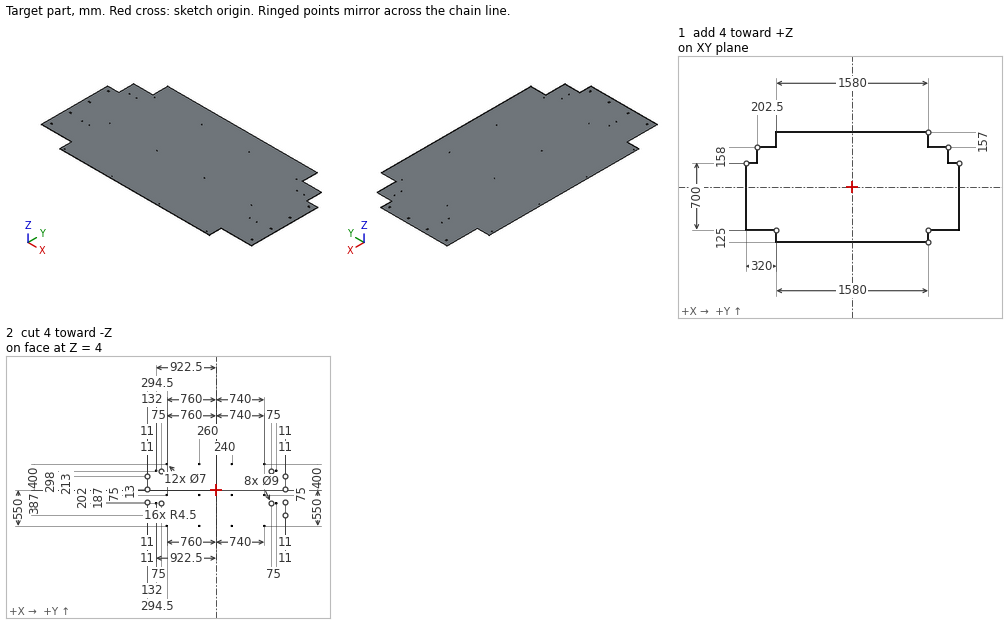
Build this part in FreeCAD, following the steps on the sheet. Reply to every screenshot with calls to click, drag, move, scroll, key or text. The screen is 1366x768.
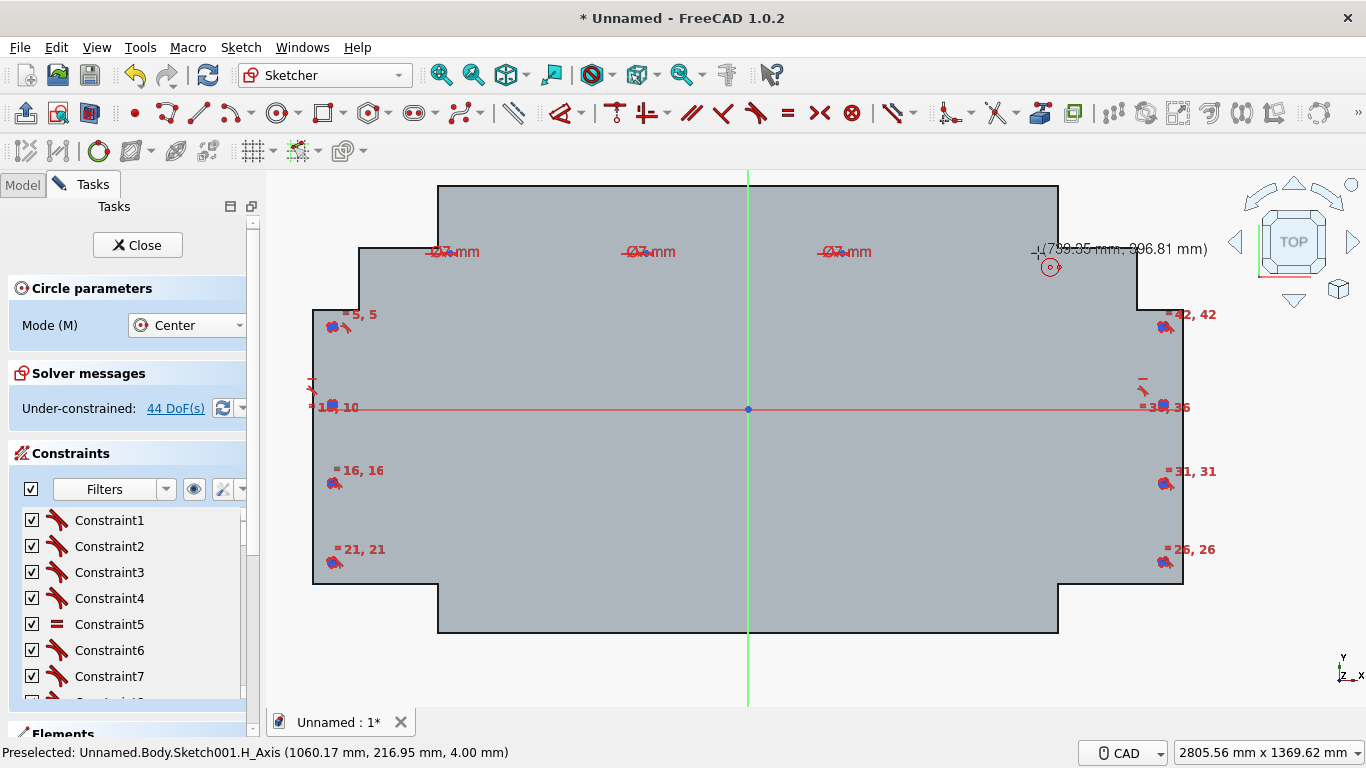
click(1038, 253)
move(1039, 252)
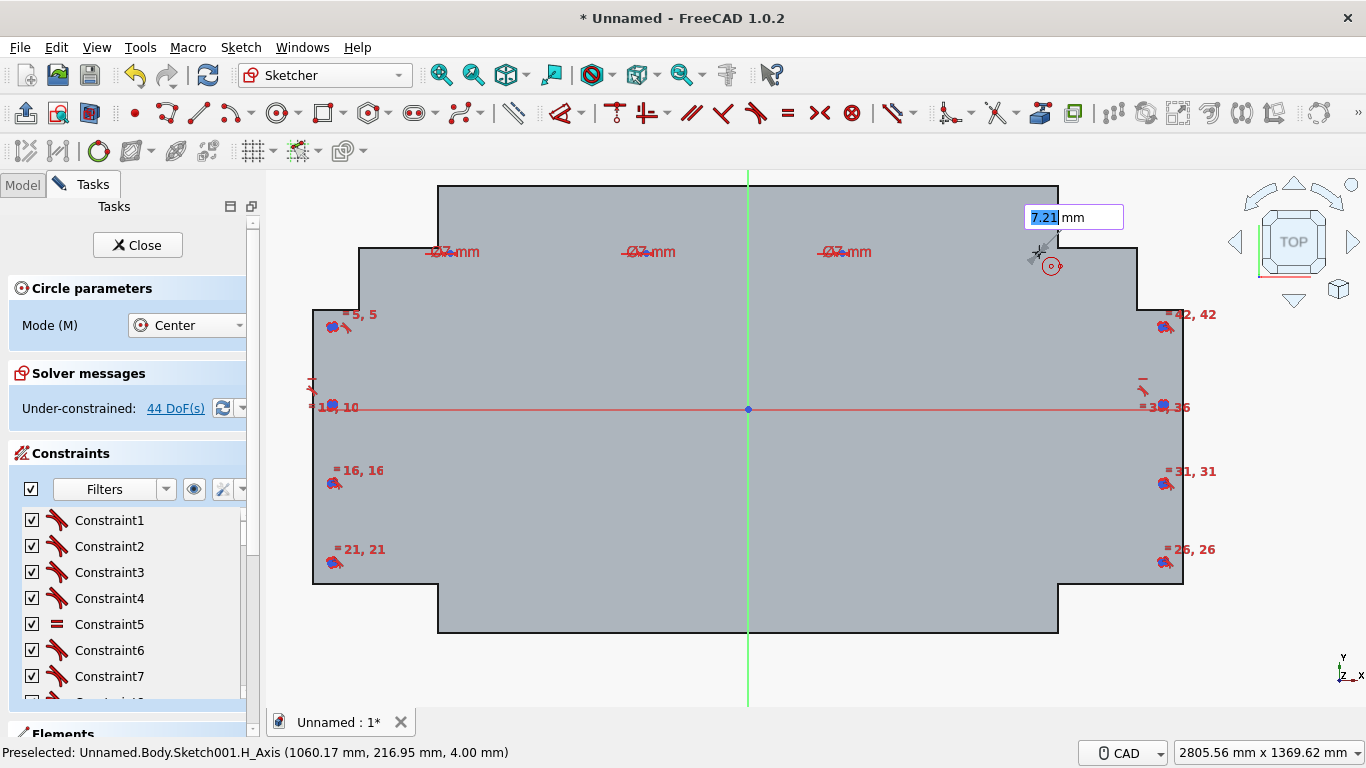
text(7)
key(Return)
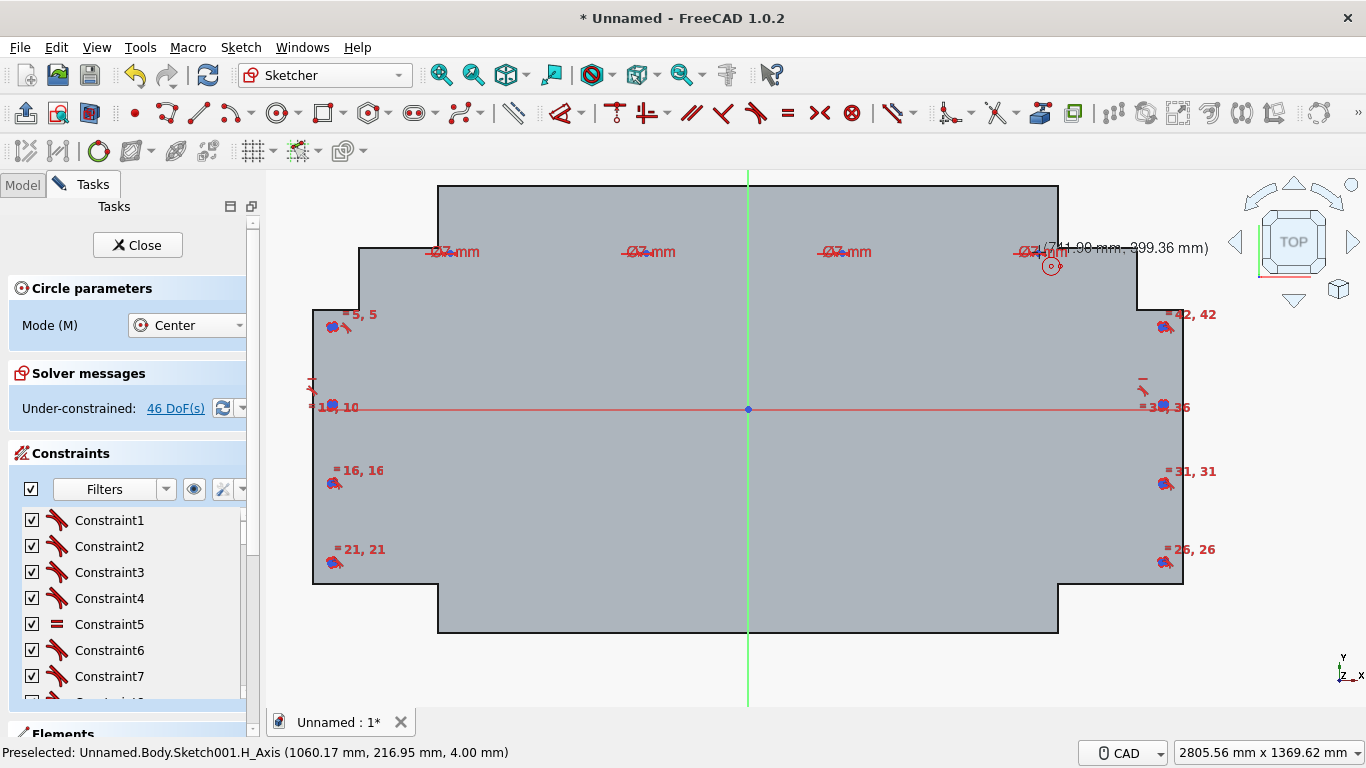
scroll(450, 439, up, 15)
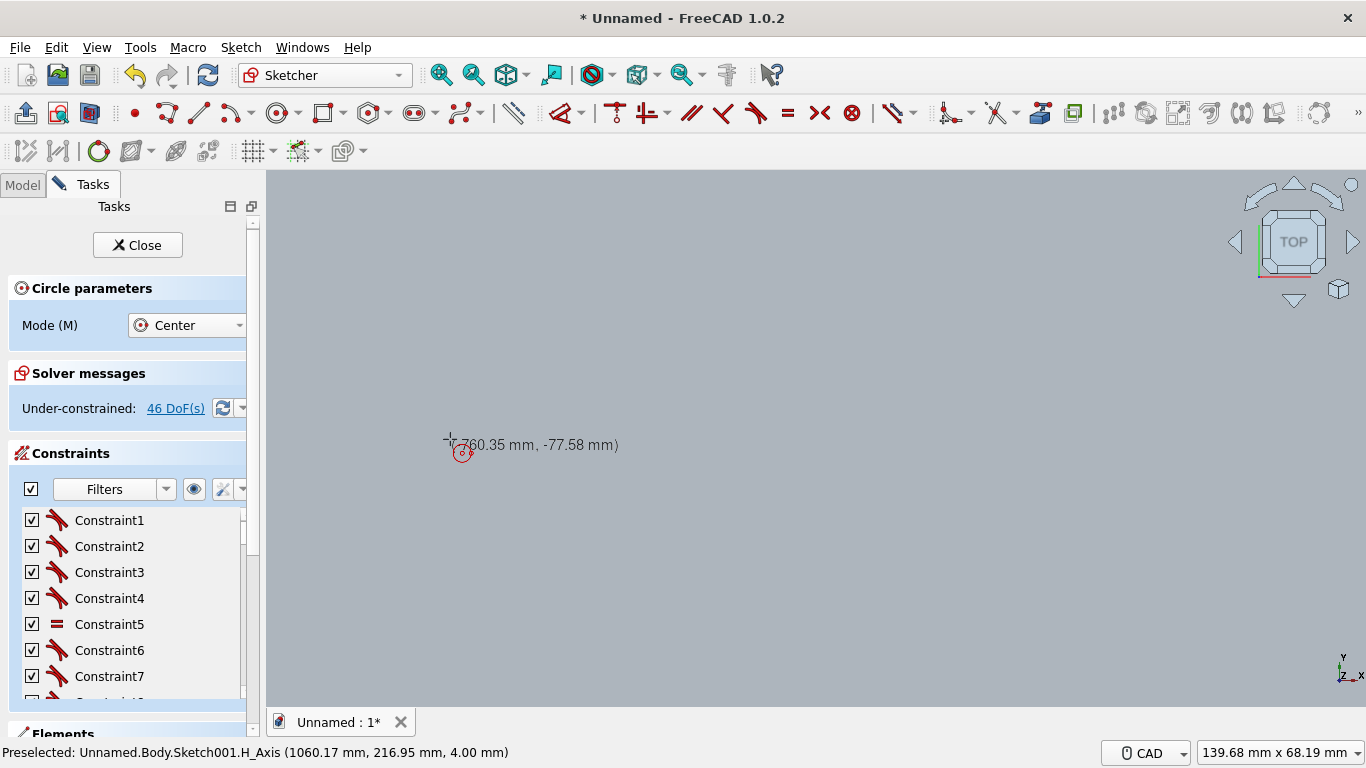
scroll(450, 439, down, 15)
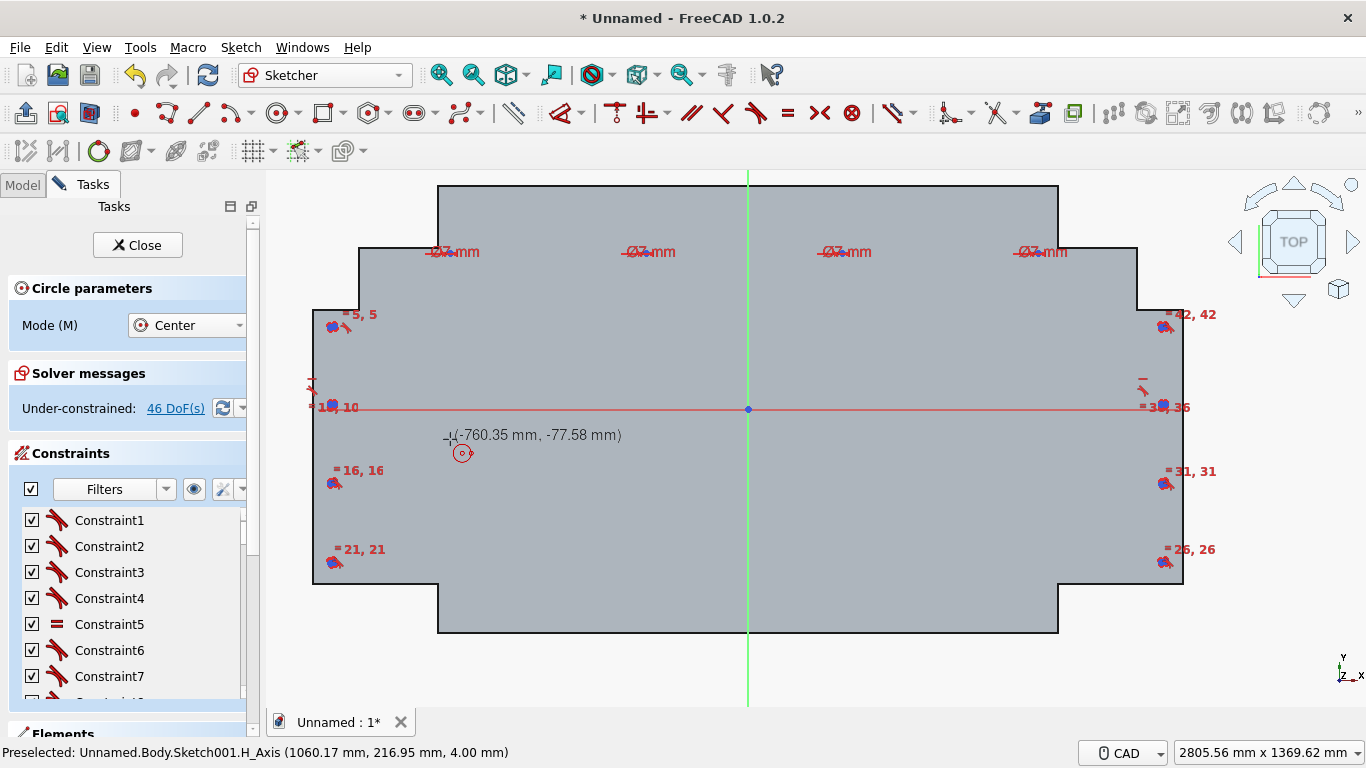
click(450, 439)
move(451, 438)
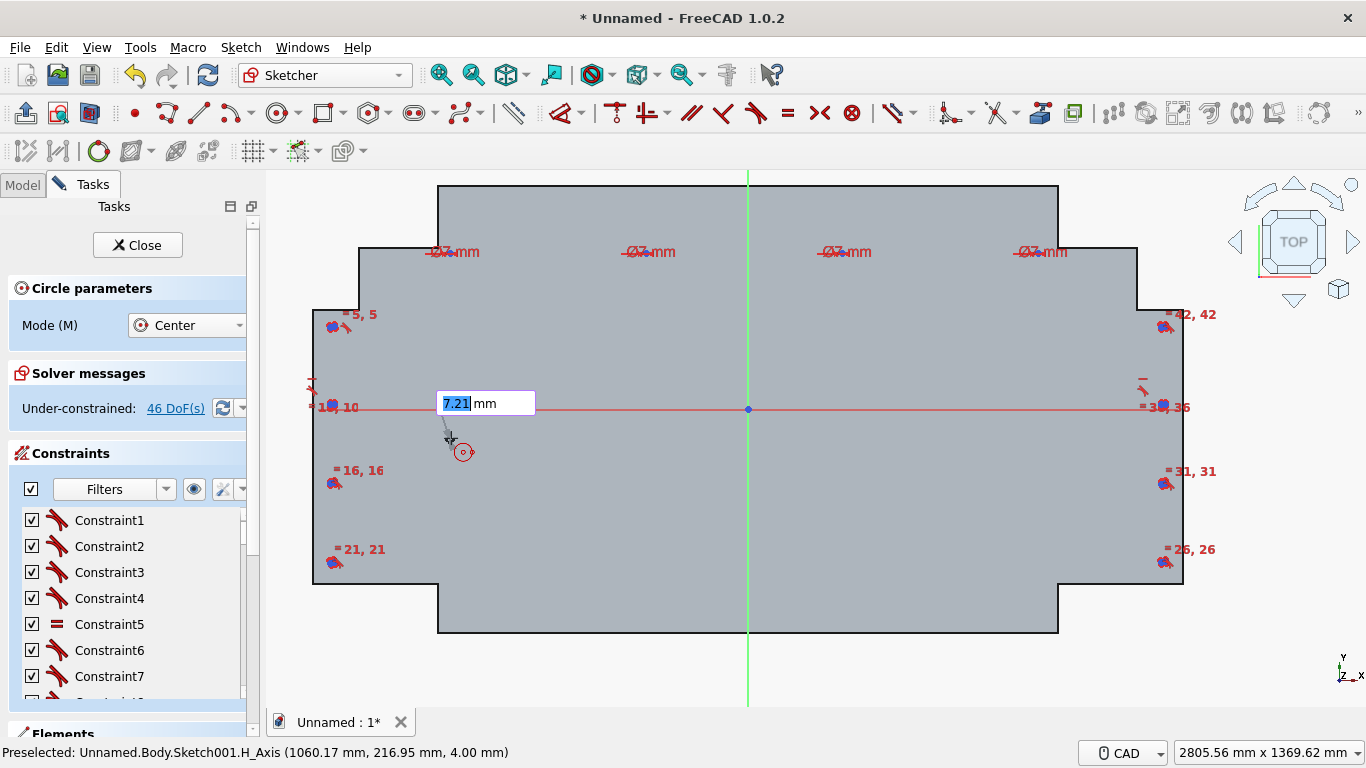
text(7)
key(Return)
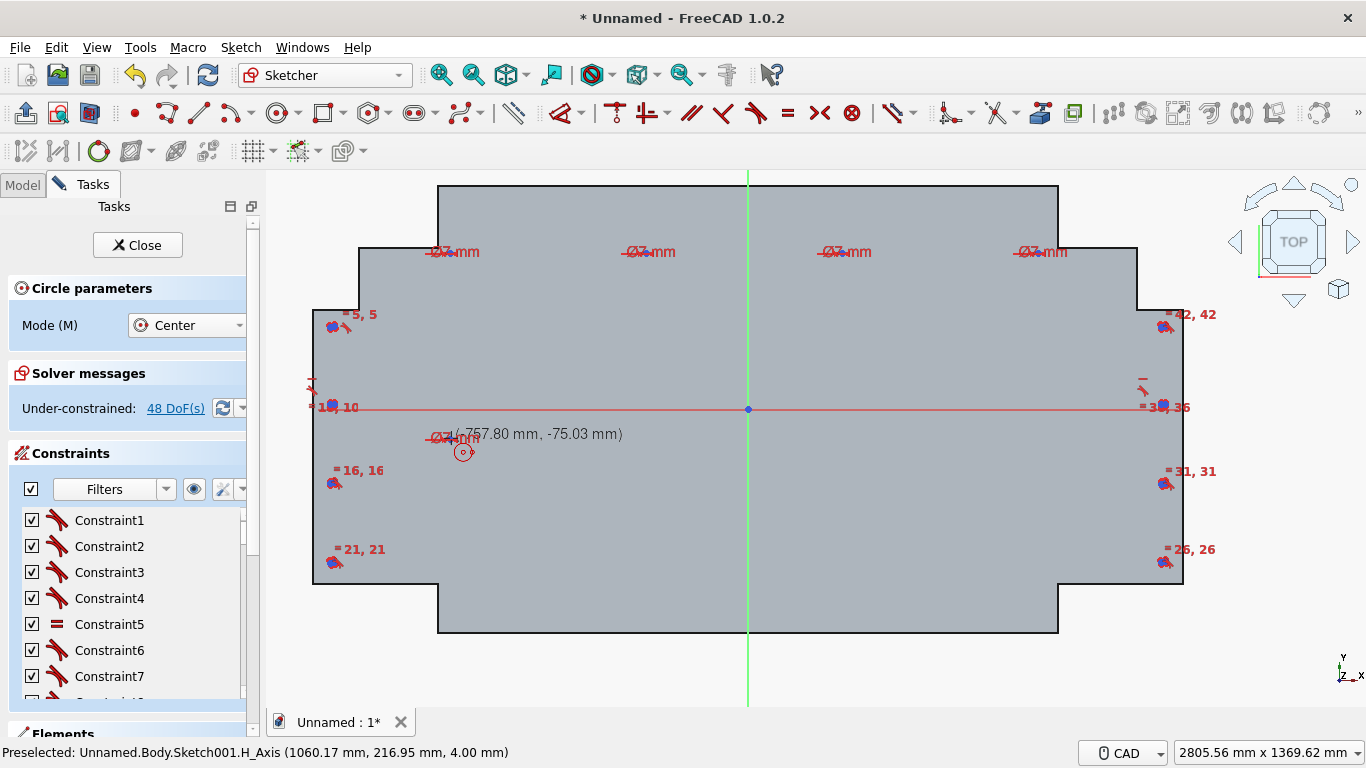
scroll(646, 439, up, 15)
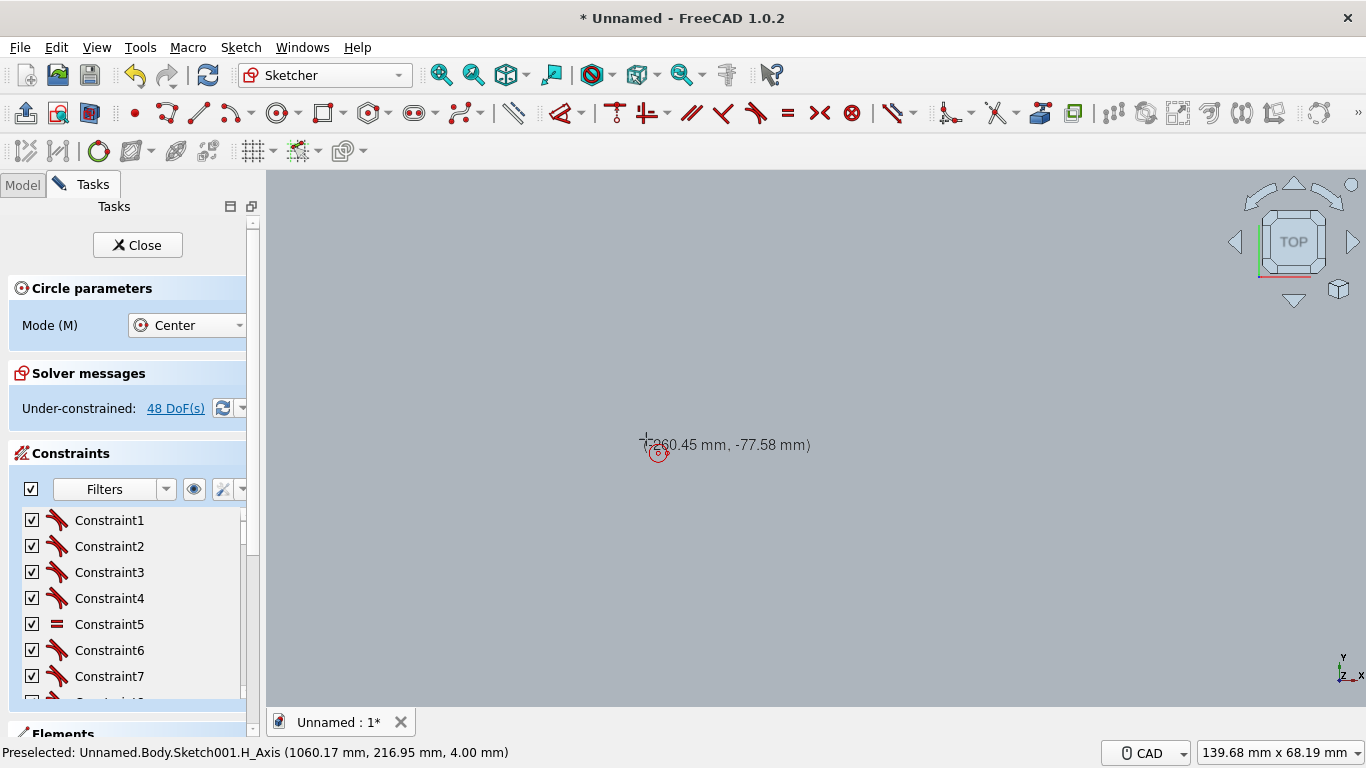
scroll(646, 439, down, 15)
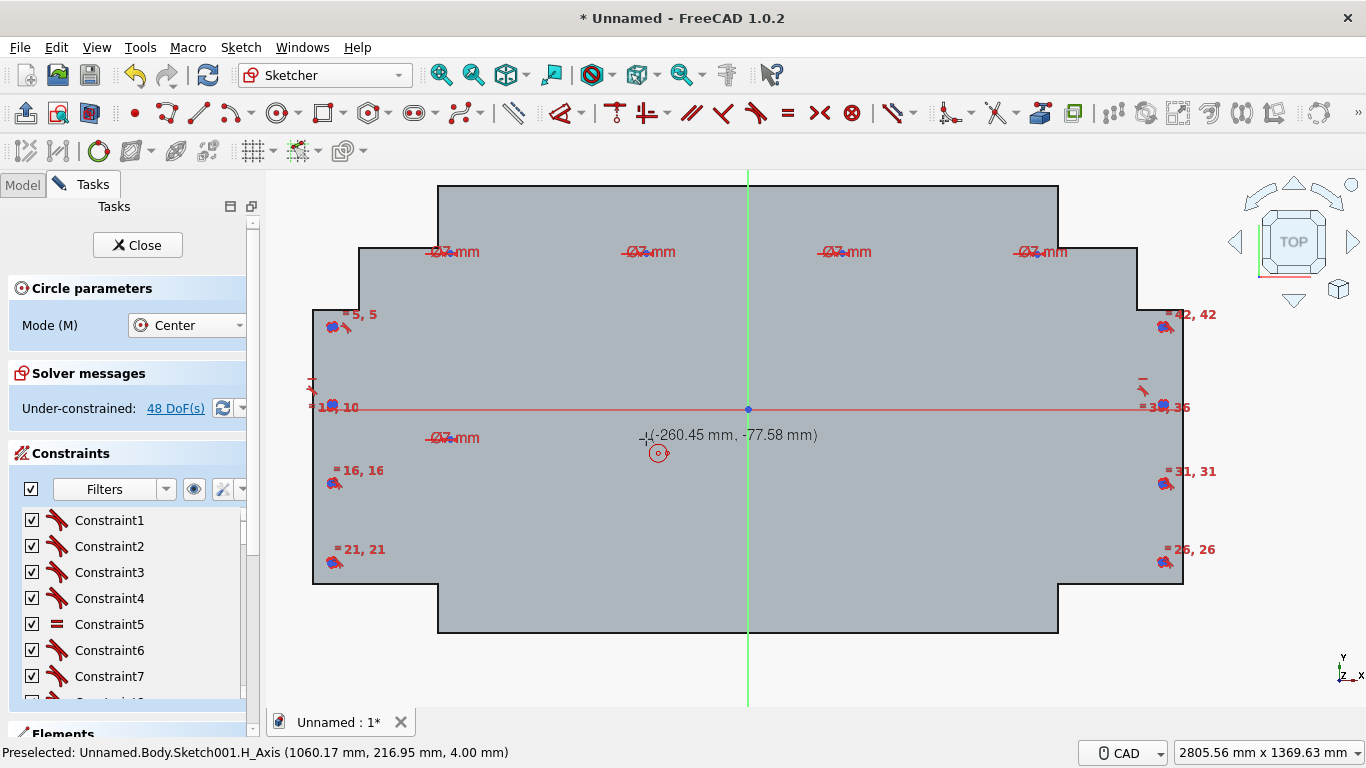
click(646, 439)
move(647, 438)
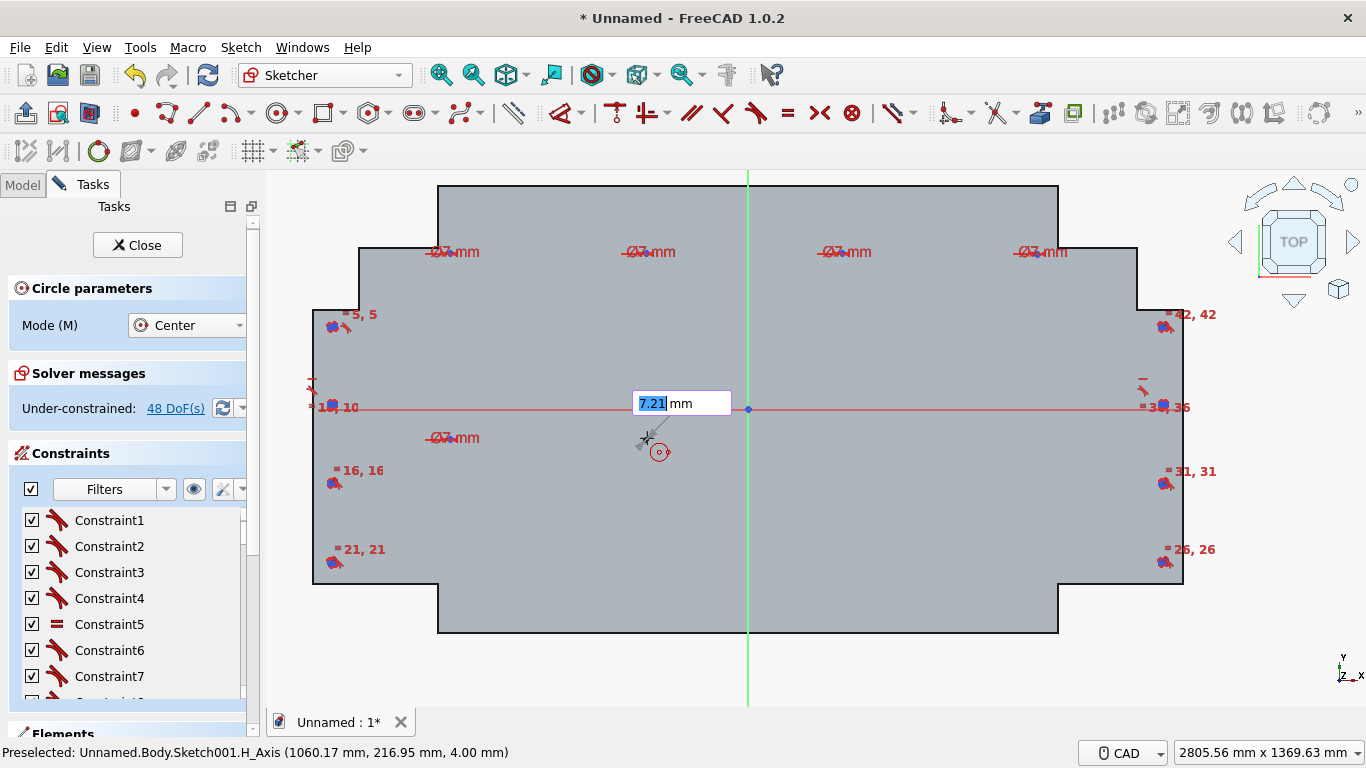
text(7)
key(Return)